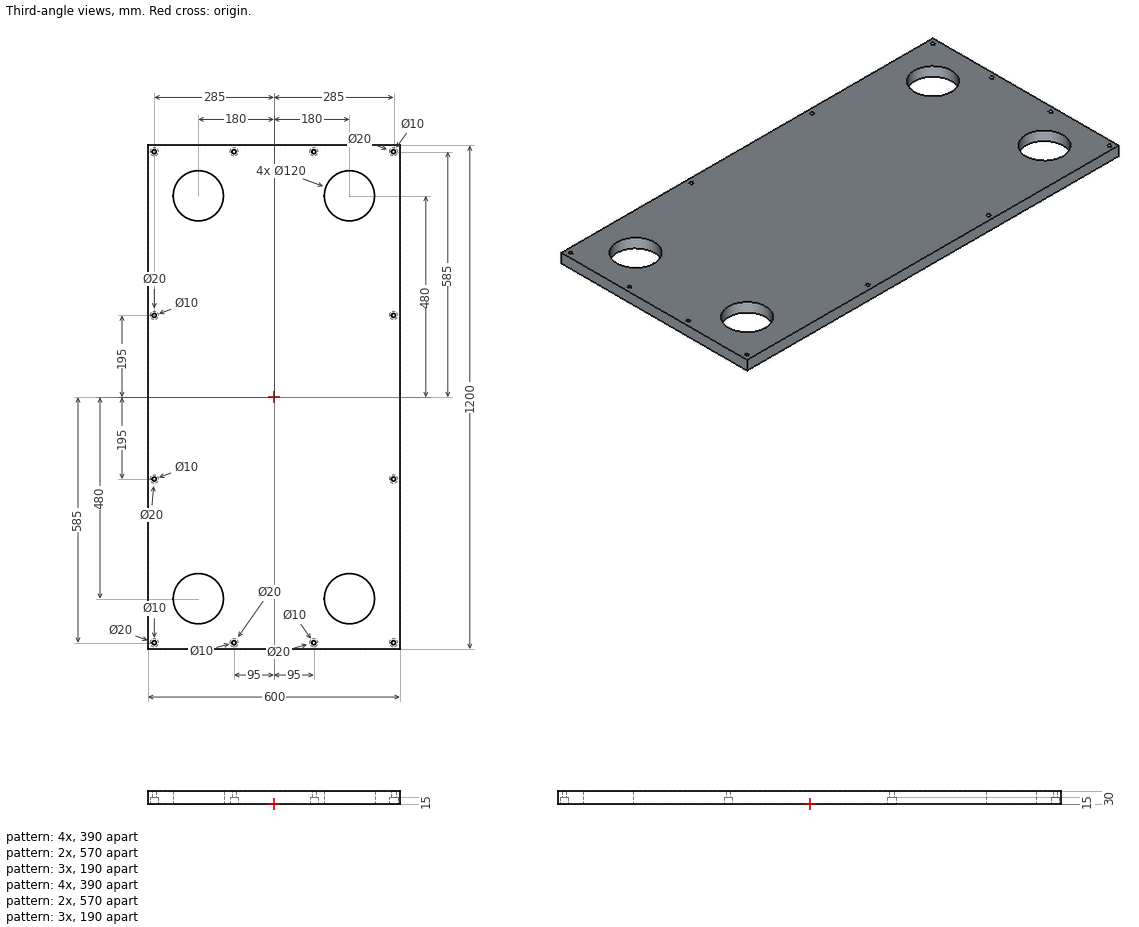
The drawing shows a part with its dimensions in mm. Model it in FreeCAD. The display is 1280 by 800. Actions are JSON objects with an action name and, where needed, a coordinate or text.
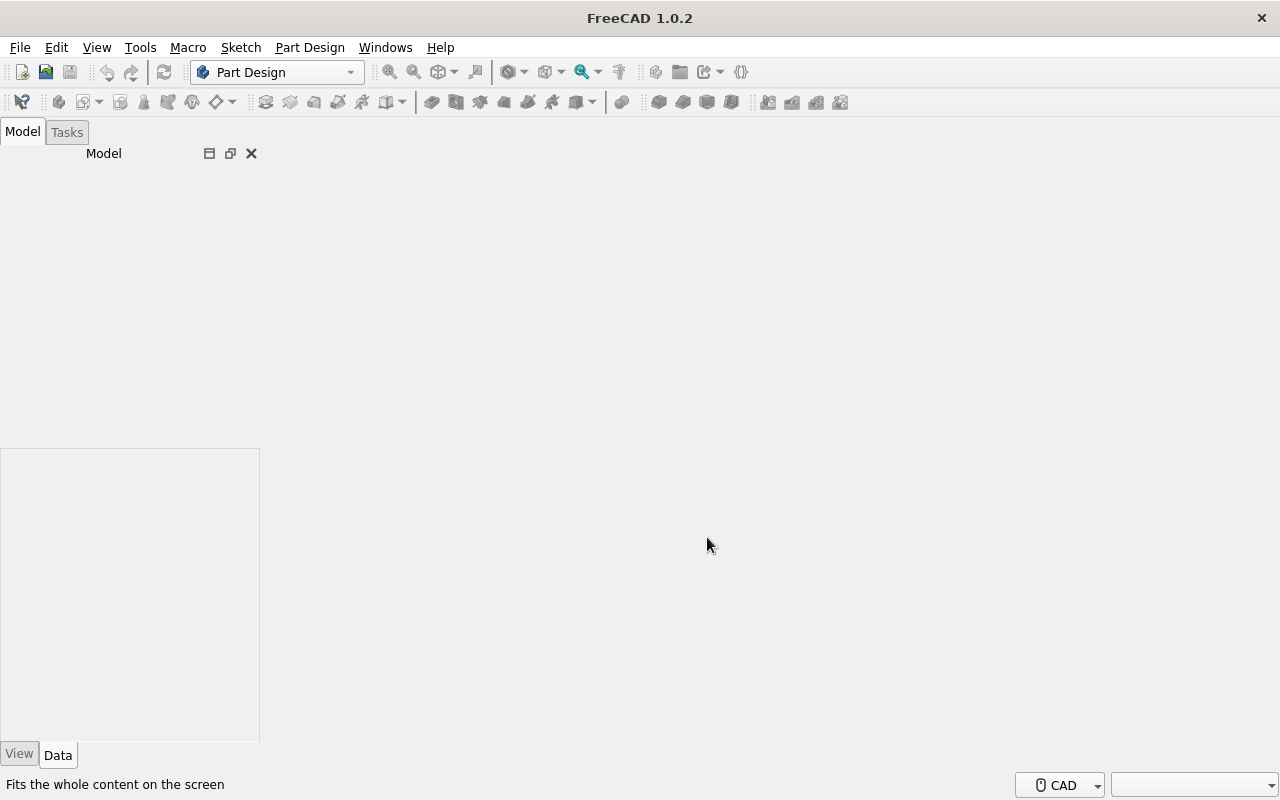
{"action": "left_click", "coordinate": [22, 72]}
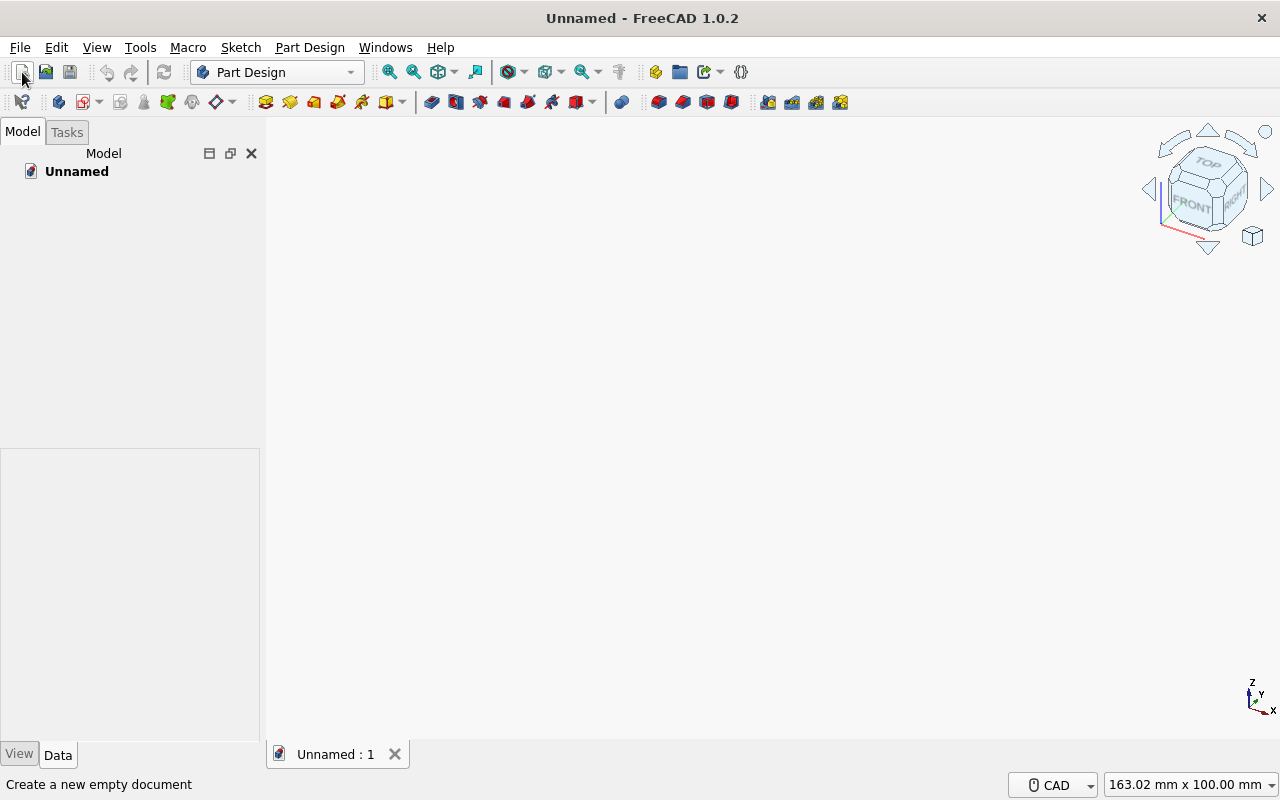
{"action": "left_click", "coordinate": [84, 102]}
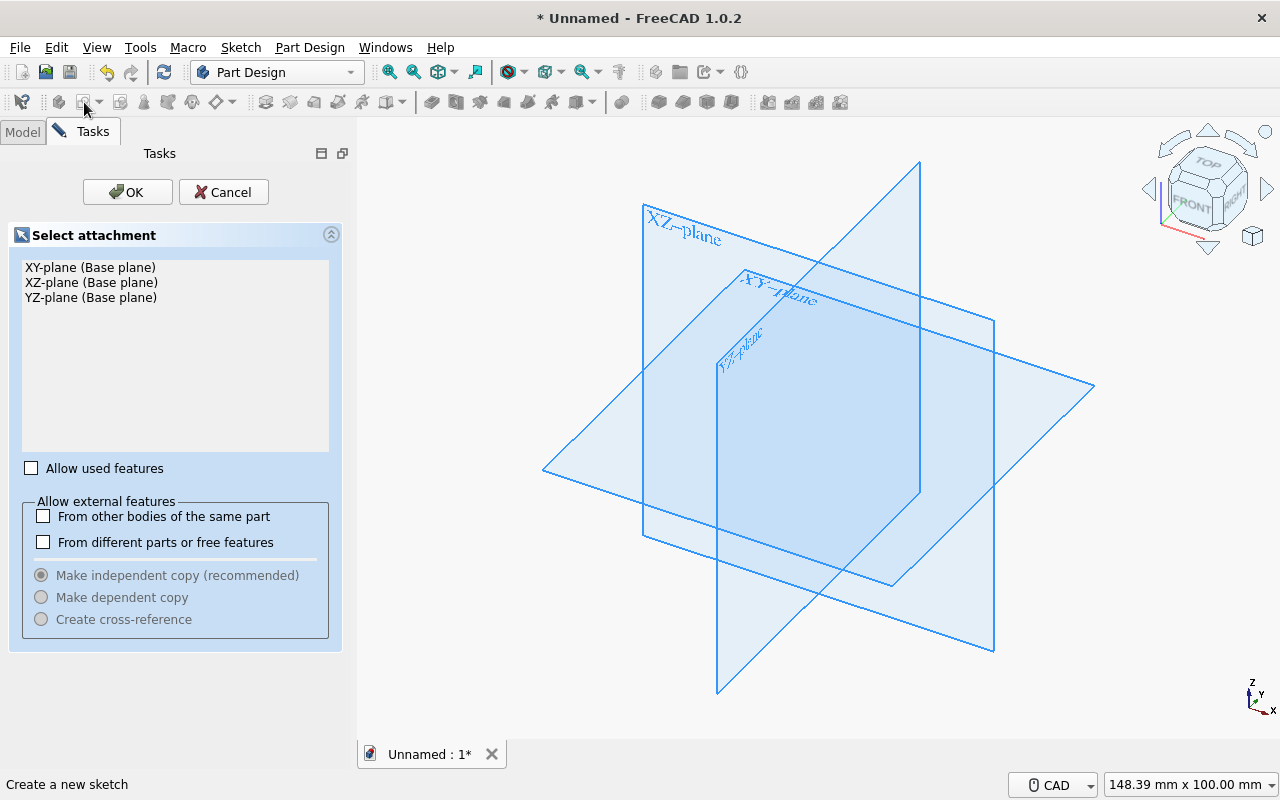
{"action": "left_click", "coordinate": [82, 268]}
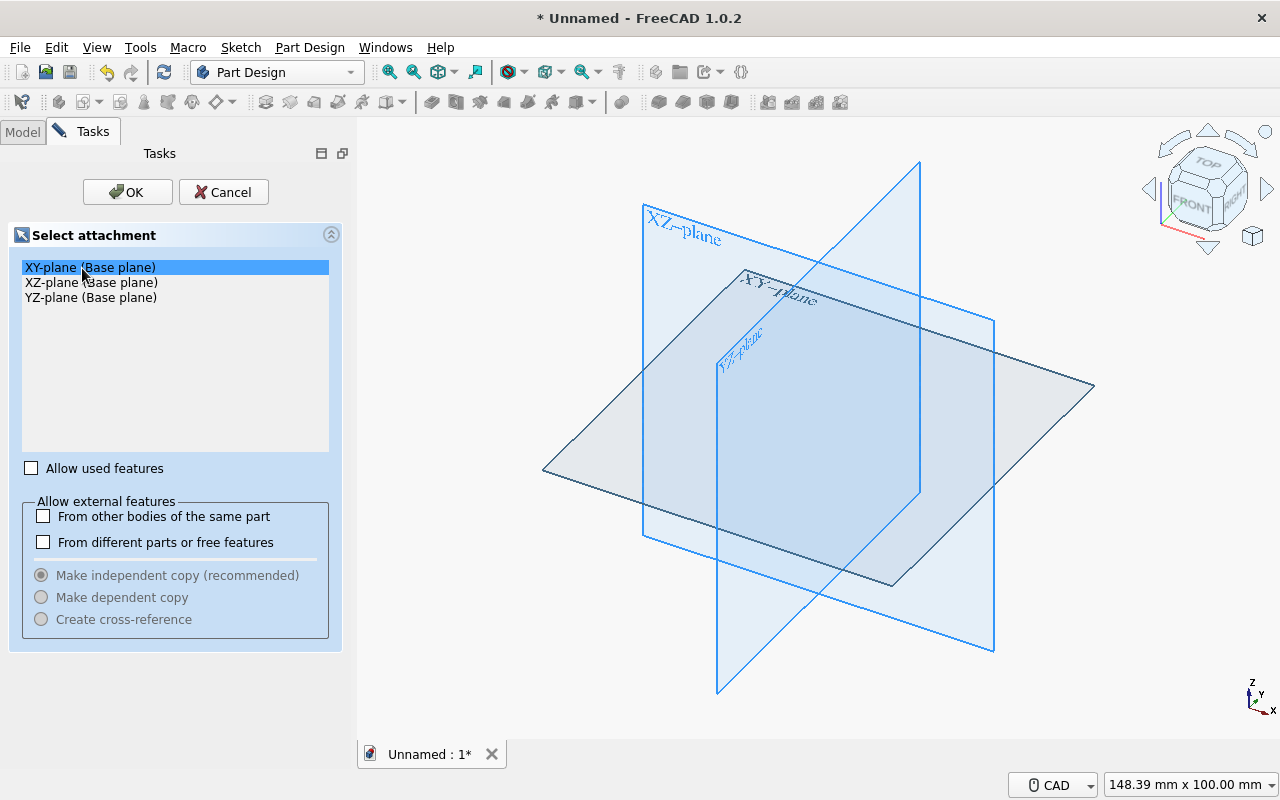
{"action": "left_click", "coordinate": [128, 192]}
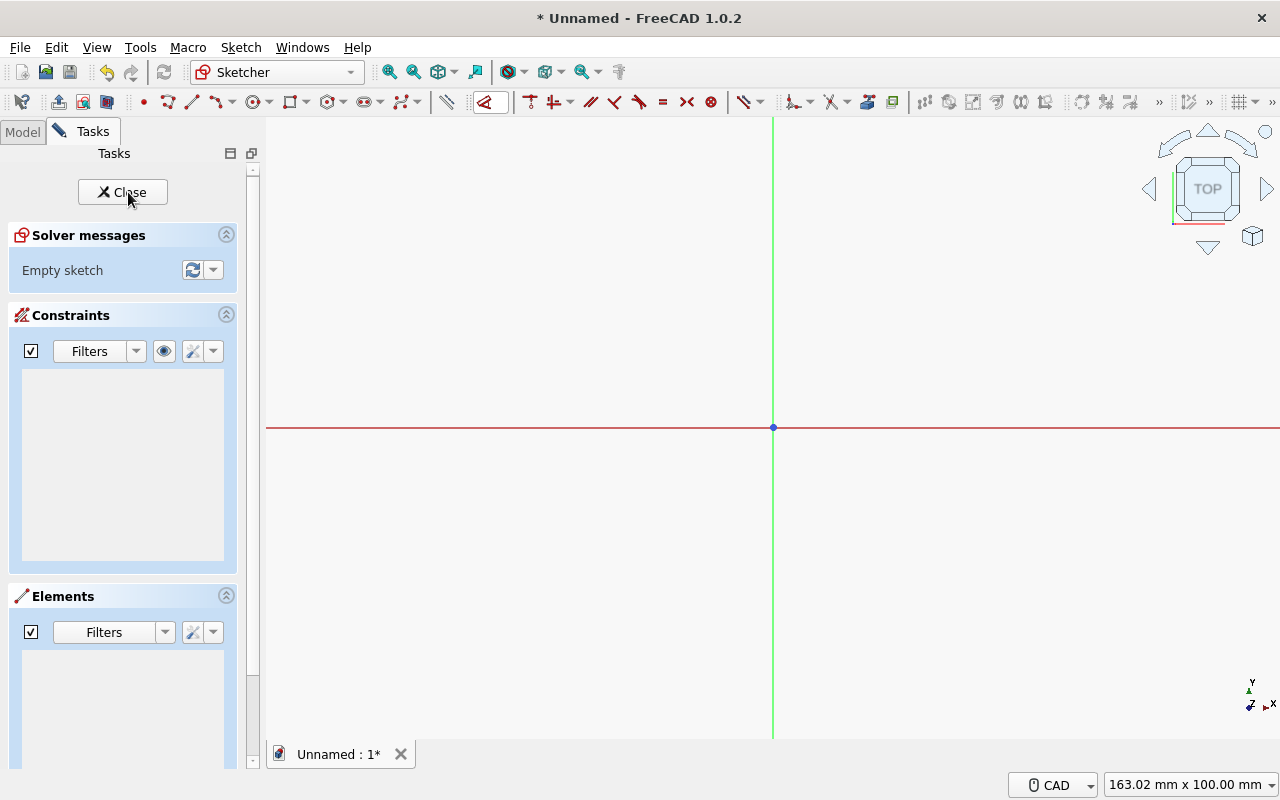
{"action": "scroll", "coordinate": [701, 428], "scroll_direction": "down", "scroll_amount": 15}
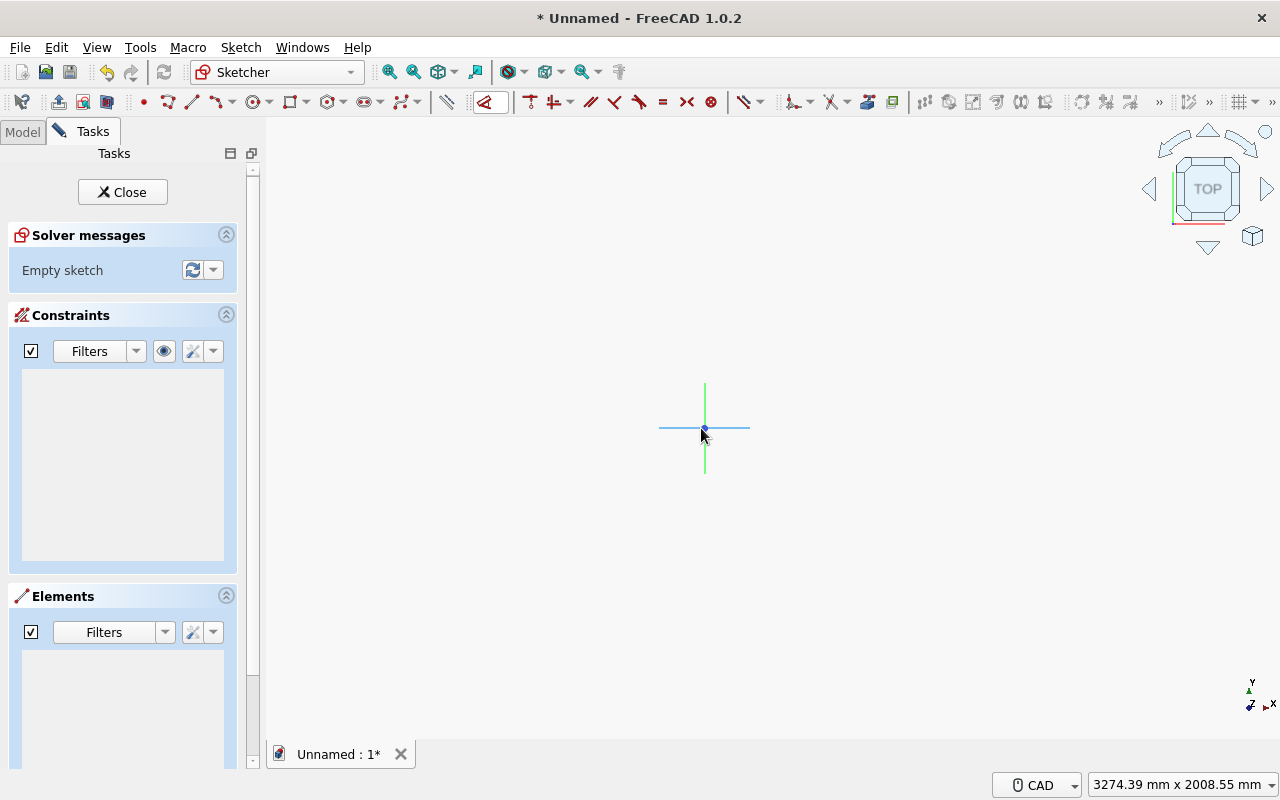
{"action": "key", "text": "g v"}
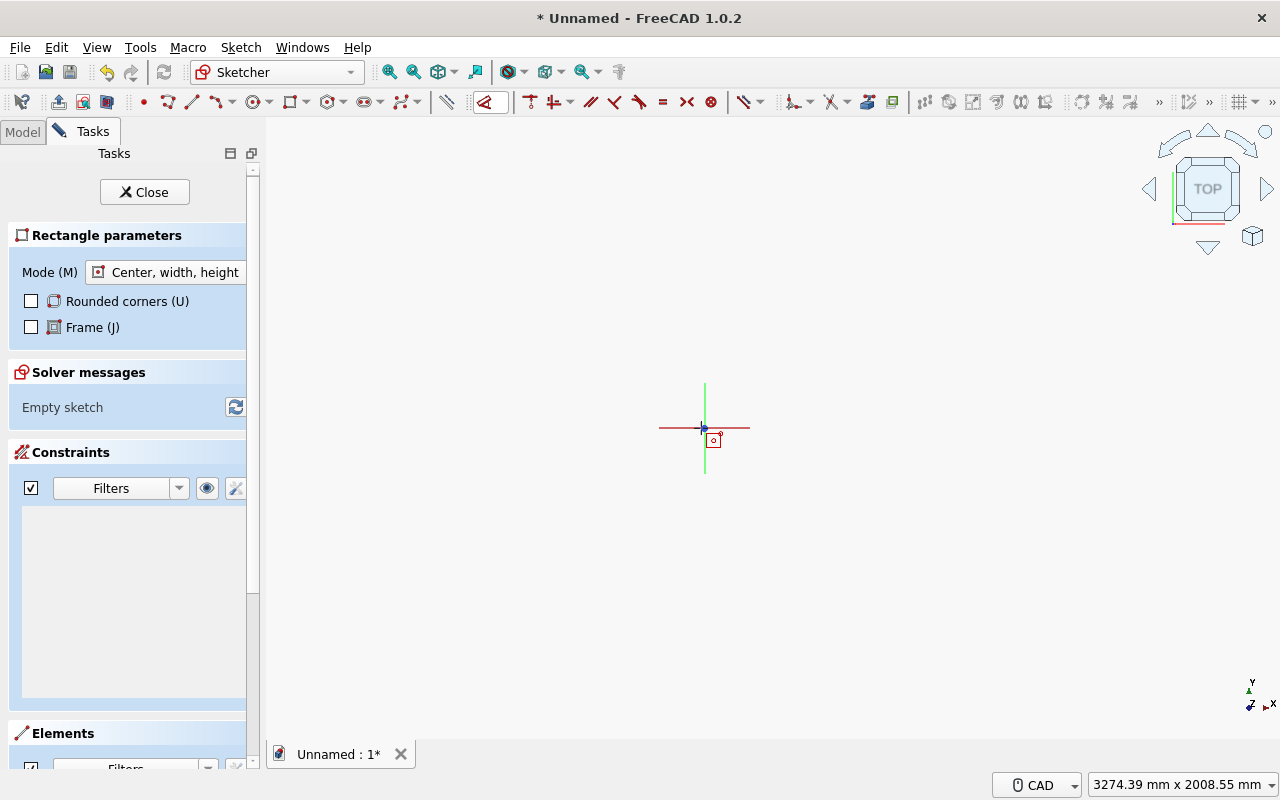
{"action": "left_click", "coordinate": [705, 428]}
{"action": "mouse_move", "coordinate": [798, 243]}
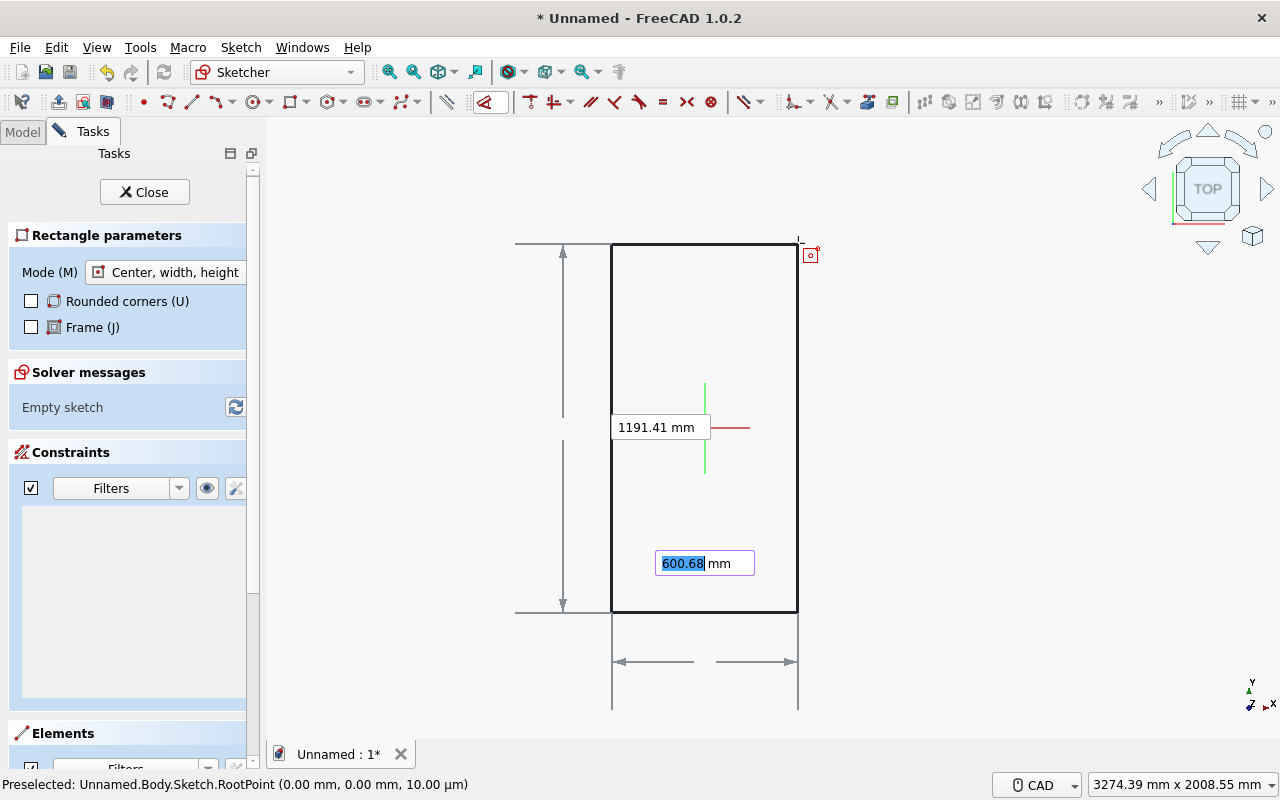
{"action": "type", "text": "600"}
{"action": "key", "text": "Tab"}
{"action": "type", "text": "1200"}
{"action": "key", "text": "Return"}
{"action": "key", "text": "Escape"}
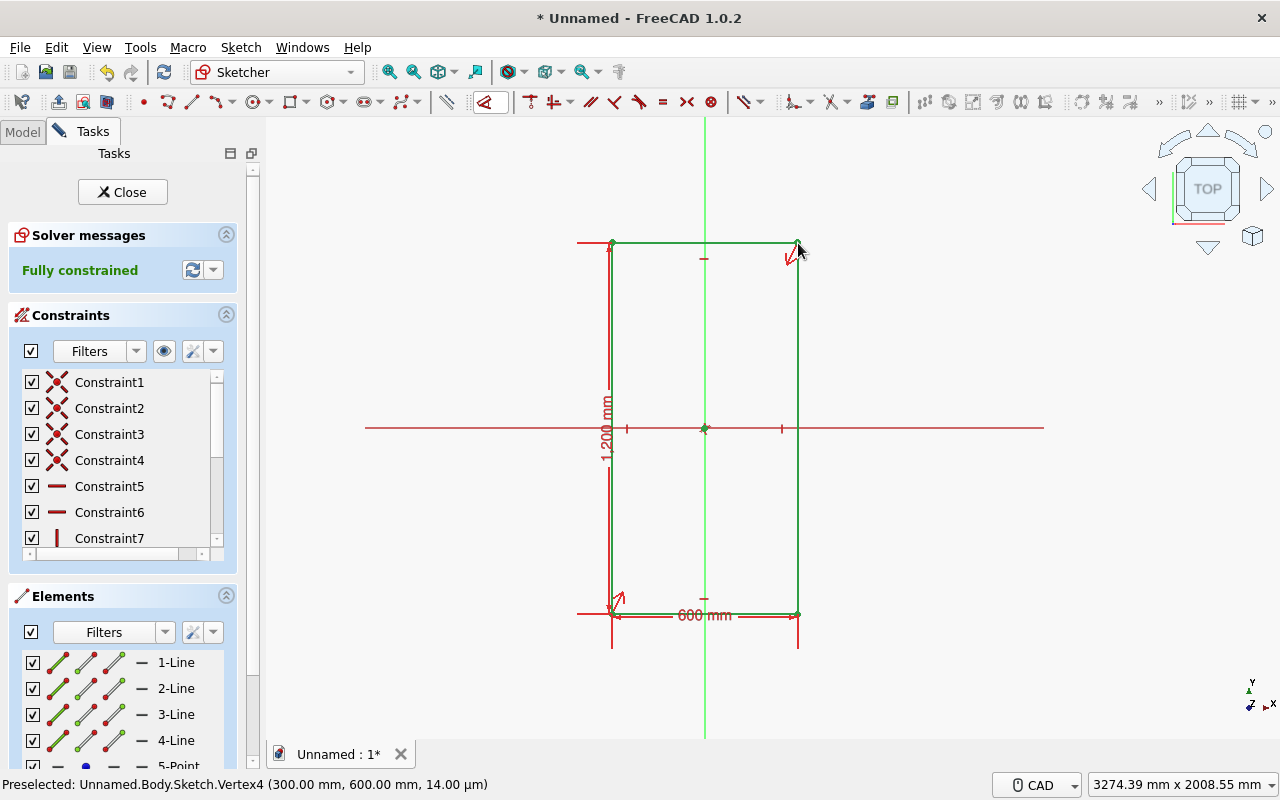
{"action": "left_click", "coordinate": [123, 192]}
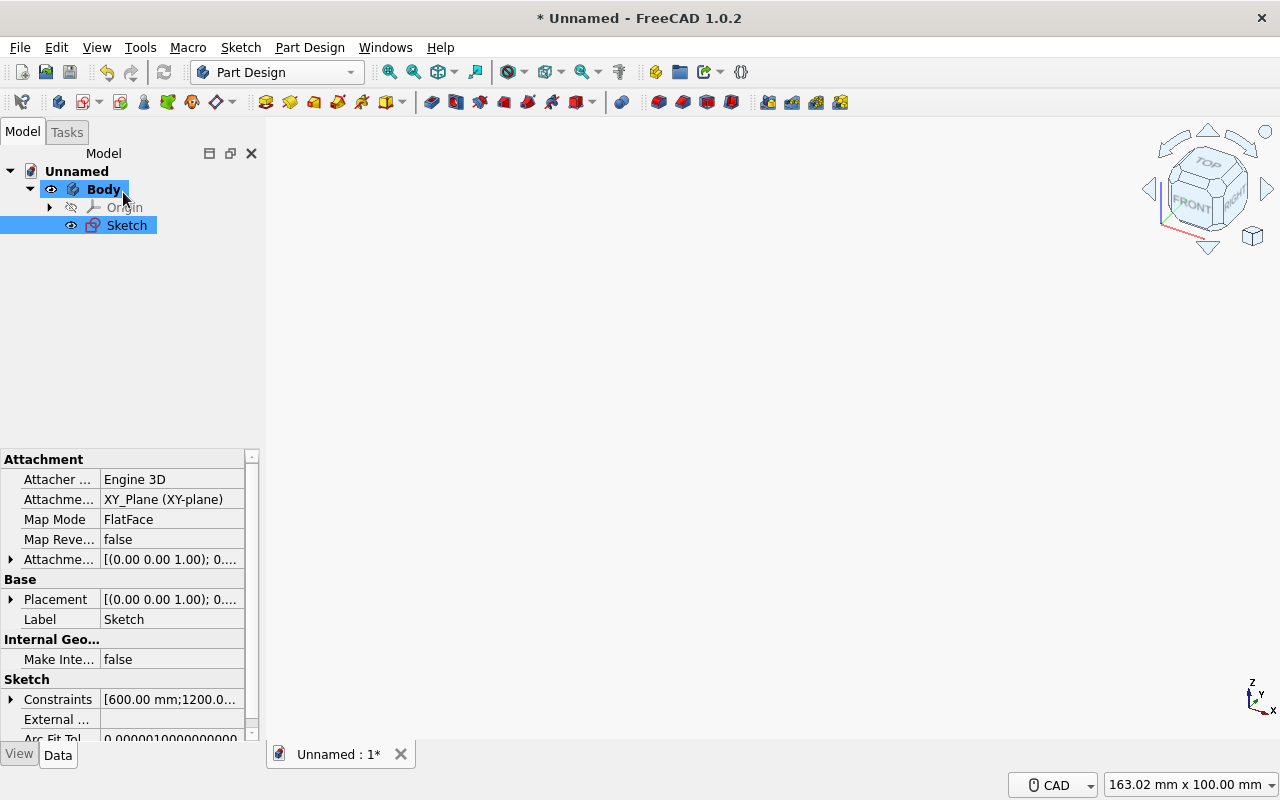
{"action": "left_click", "coordinate": [266, 102]}